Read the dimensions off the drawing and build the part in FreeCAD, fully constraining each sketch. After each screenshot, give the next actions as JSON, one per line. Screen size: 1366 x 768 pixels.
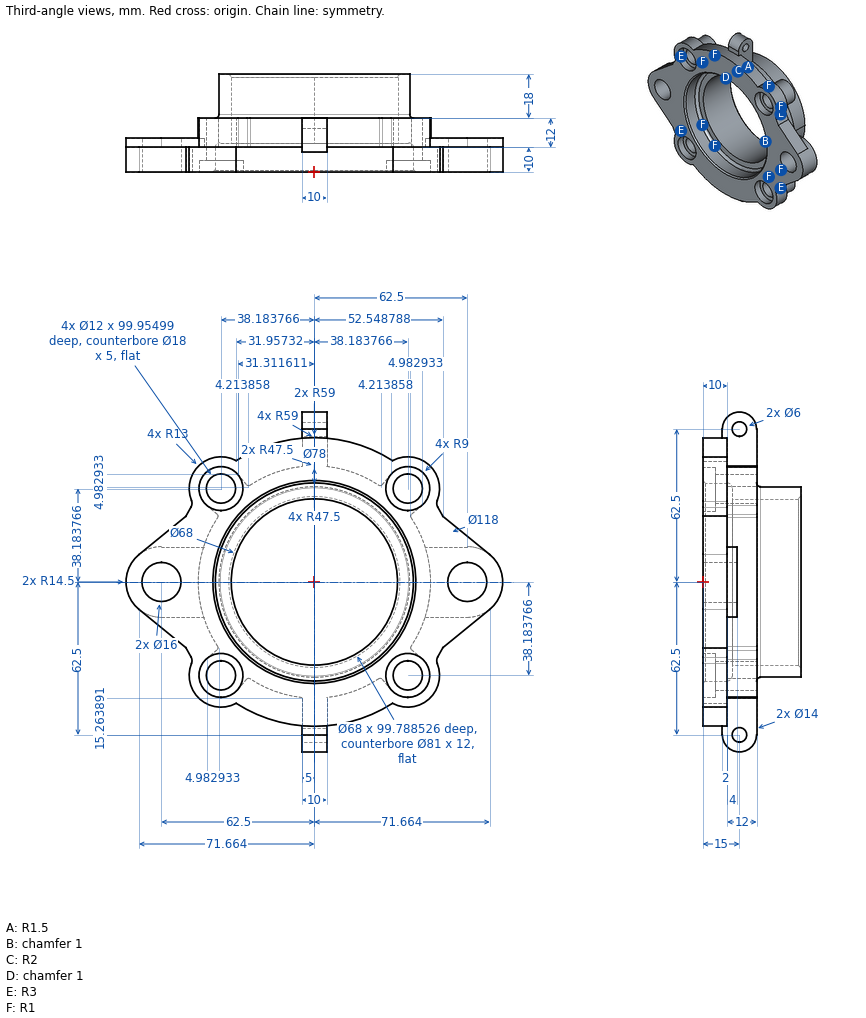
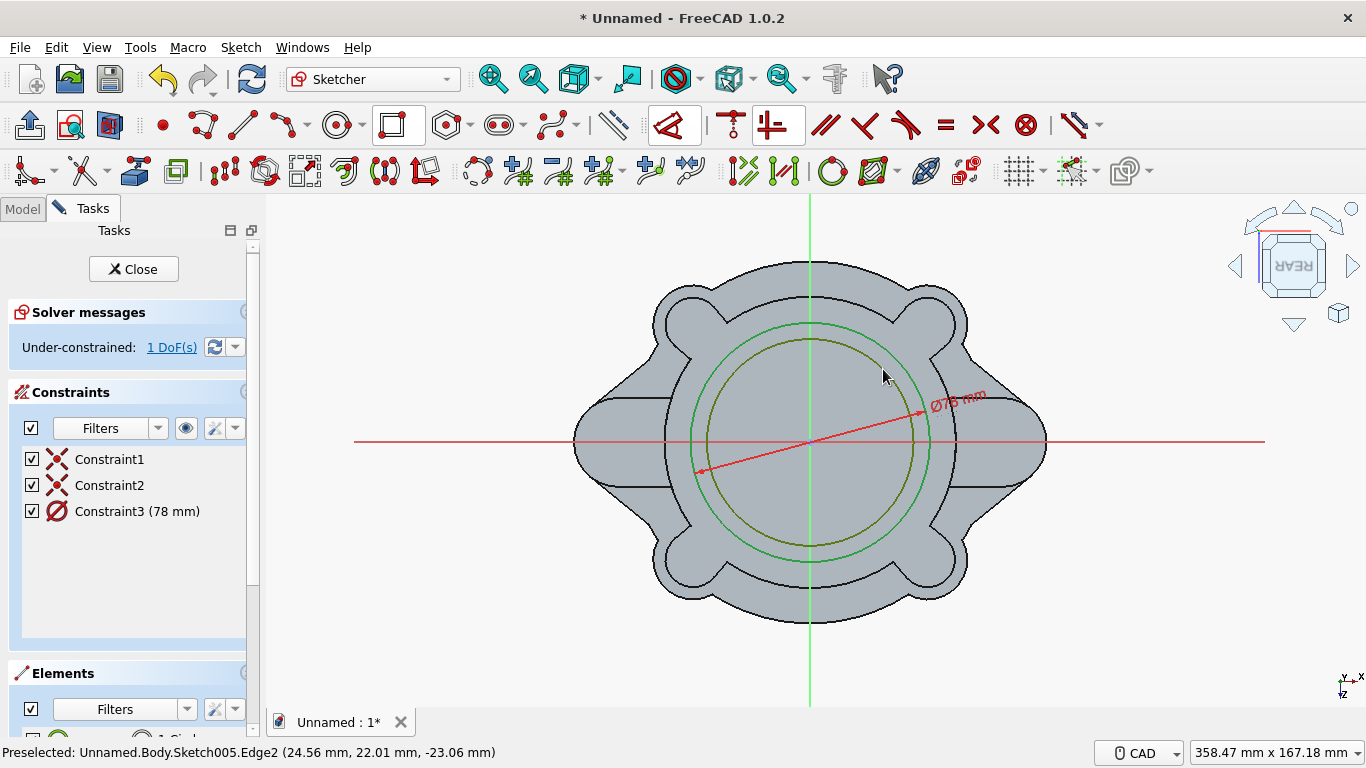
{"action": "left_click", "coordinate": [696, 126]}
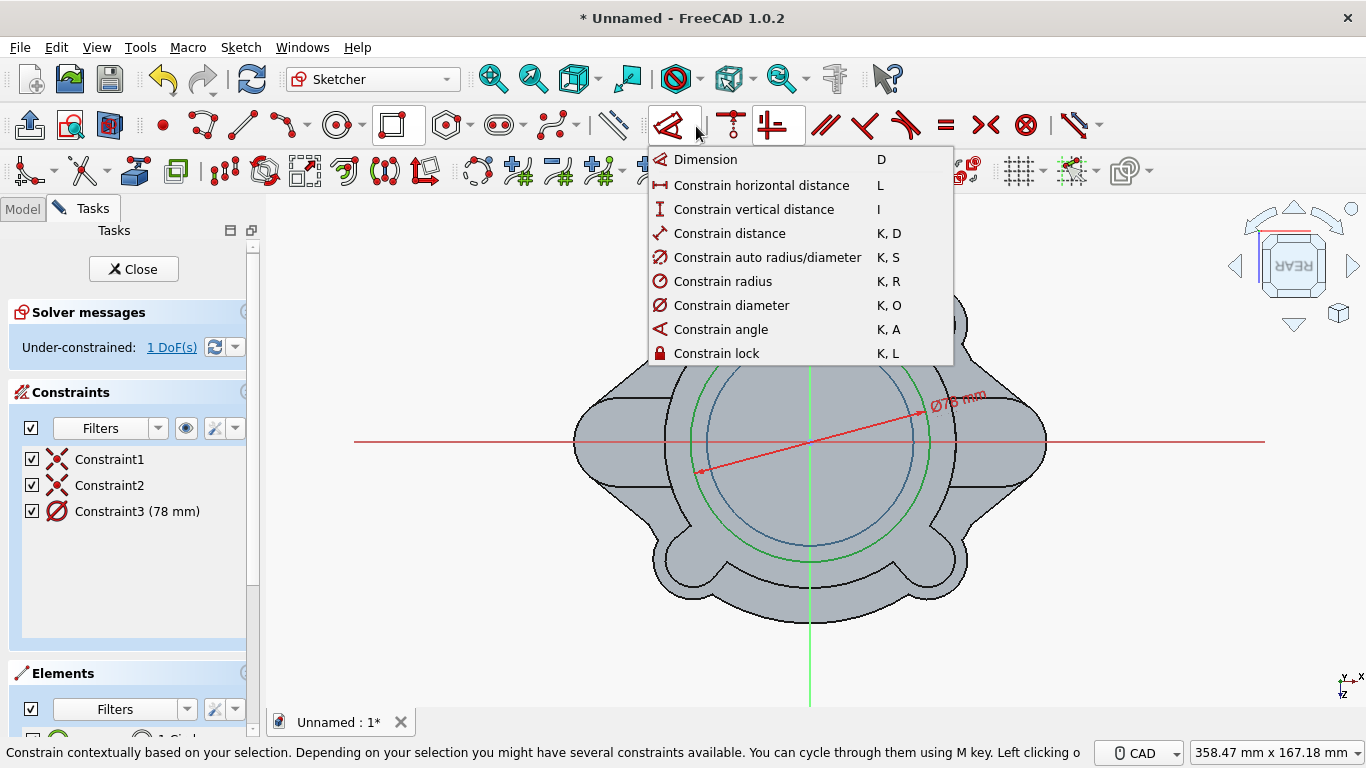
{"action": "left_click", "coordinate": [801, 305]}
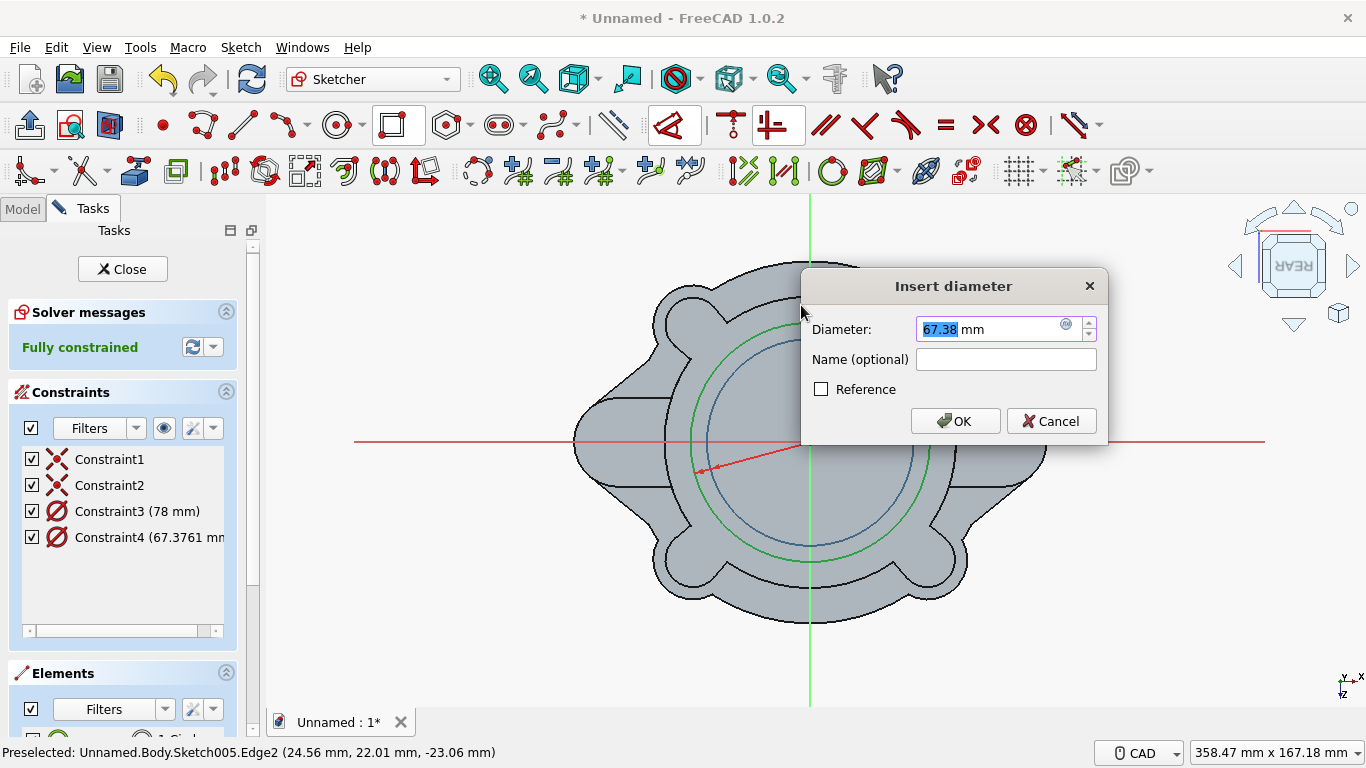
{"action": "type", "text": "68"}
{"action": "key", "text": "Return"}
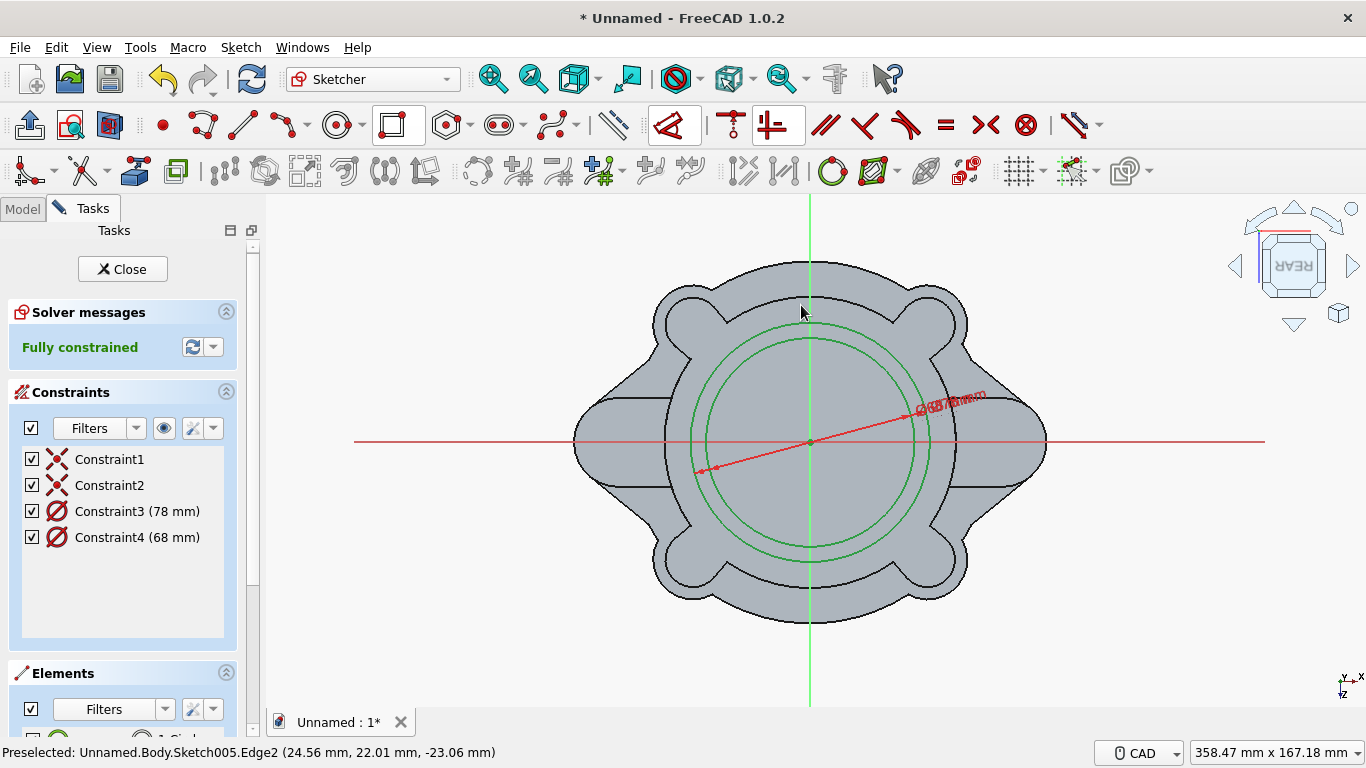
{"action": "left_click", "coordinate": [123, 269]}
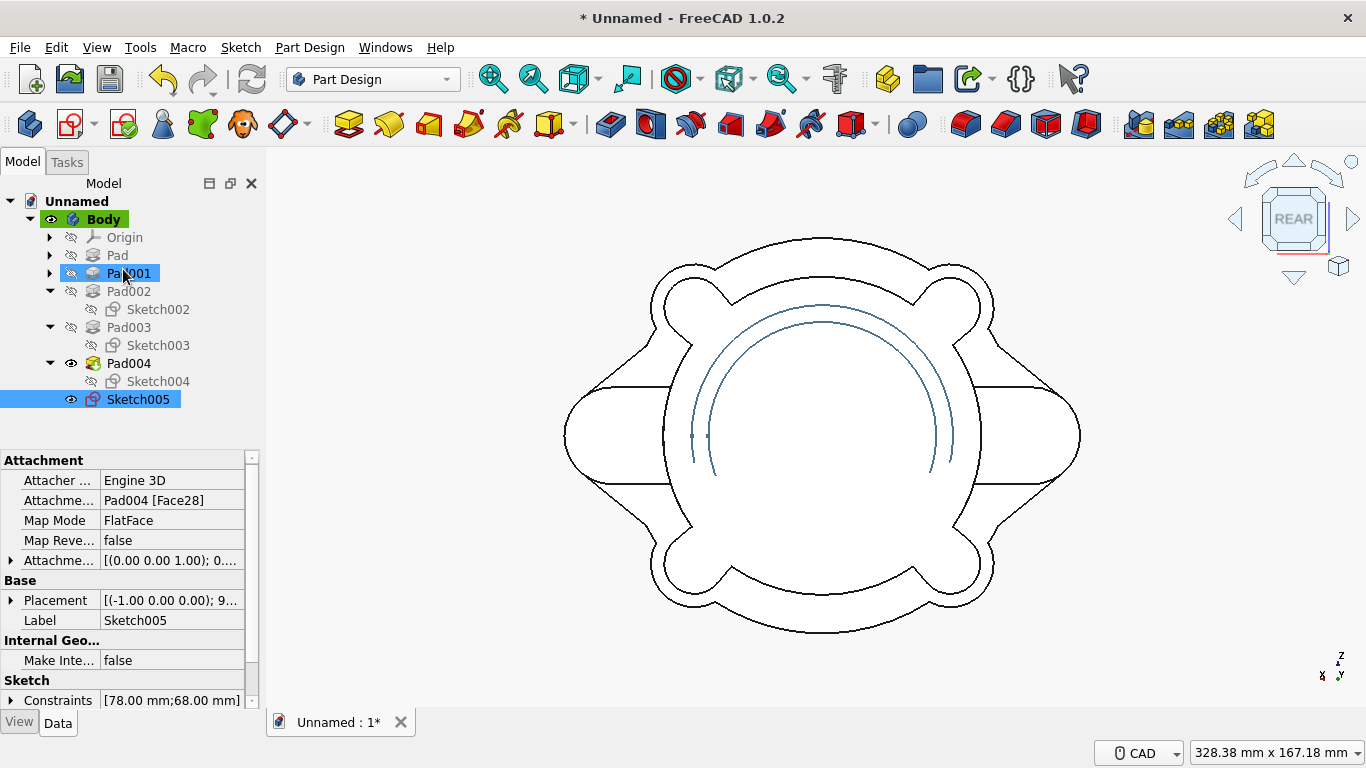
{"action": "left_click", "coordinate": [350, 124]}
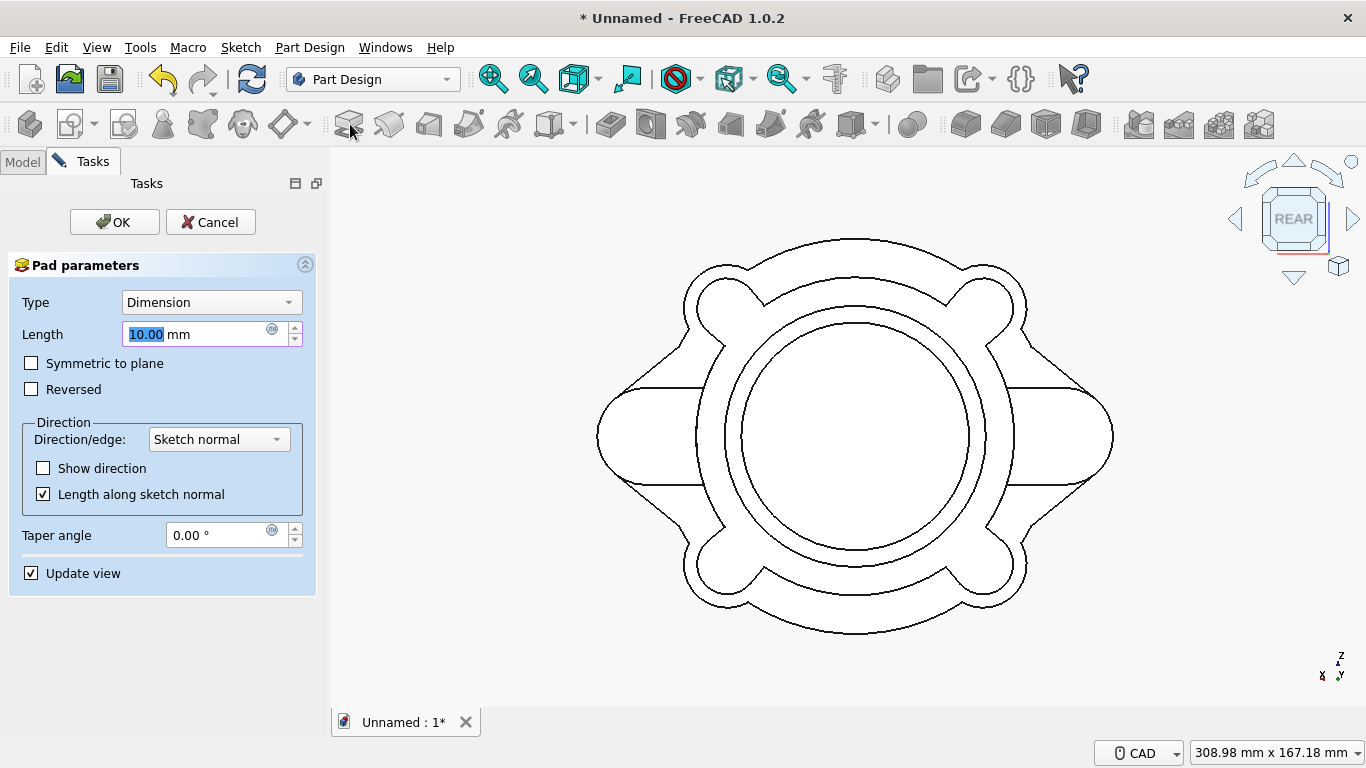
{"action": "type", "text": "18"}
{"action": "key", "text": "Tab"}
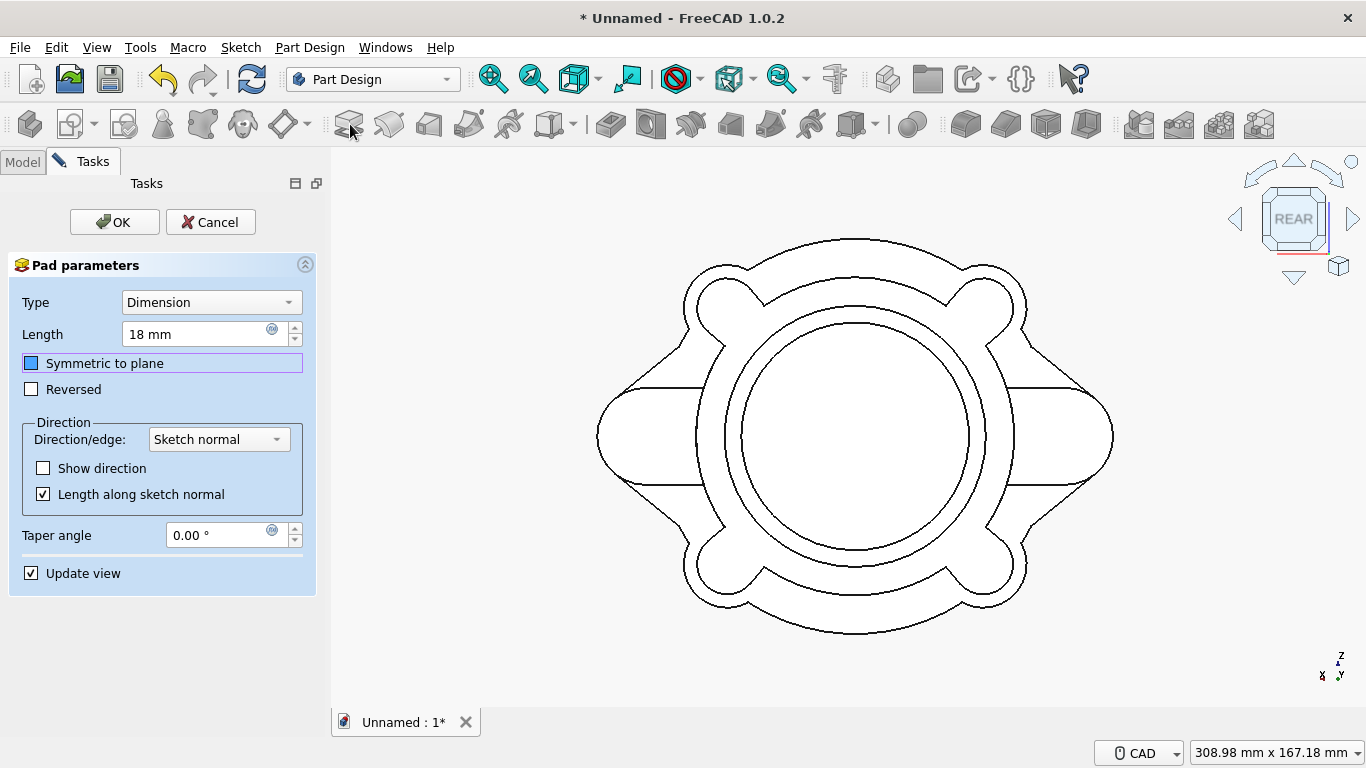
{"action": "left_click", "coordinate": [115, 222]}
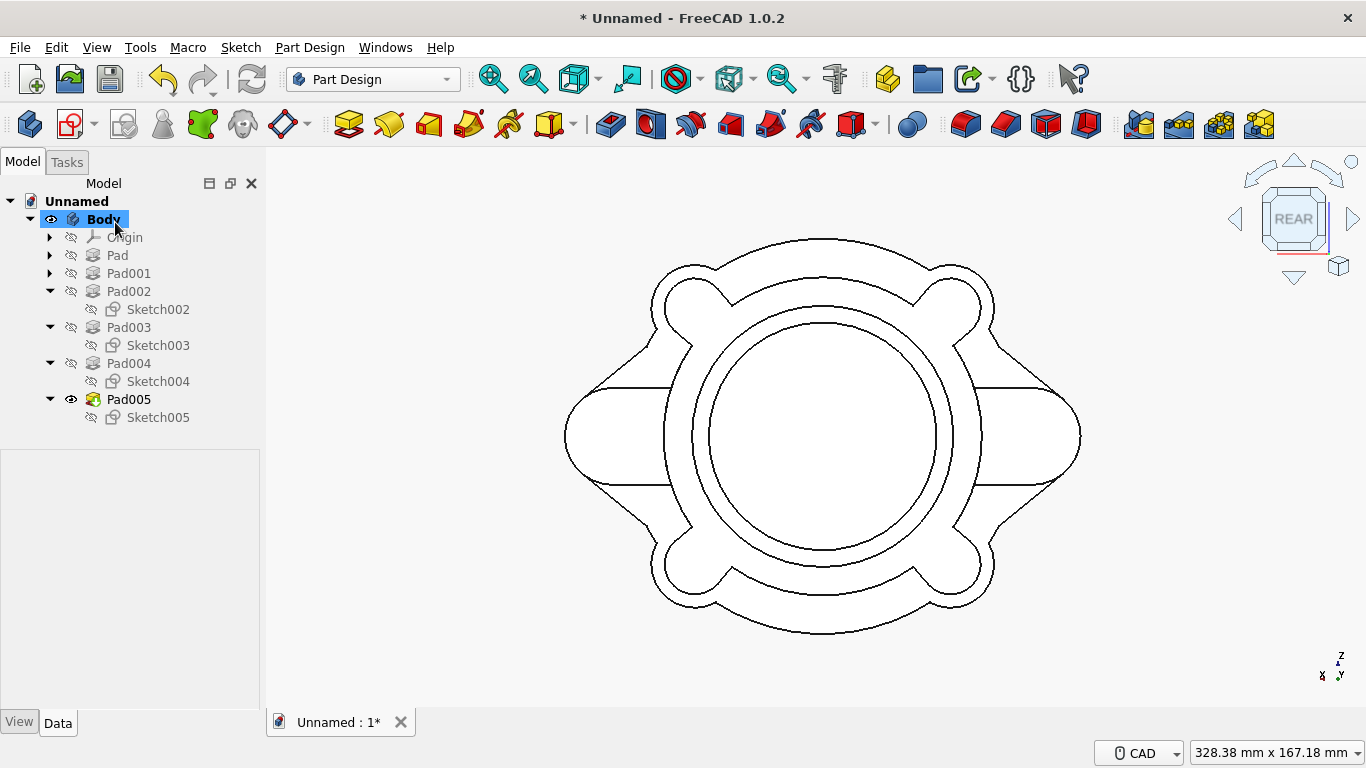
{"action": "key", "text": "0"}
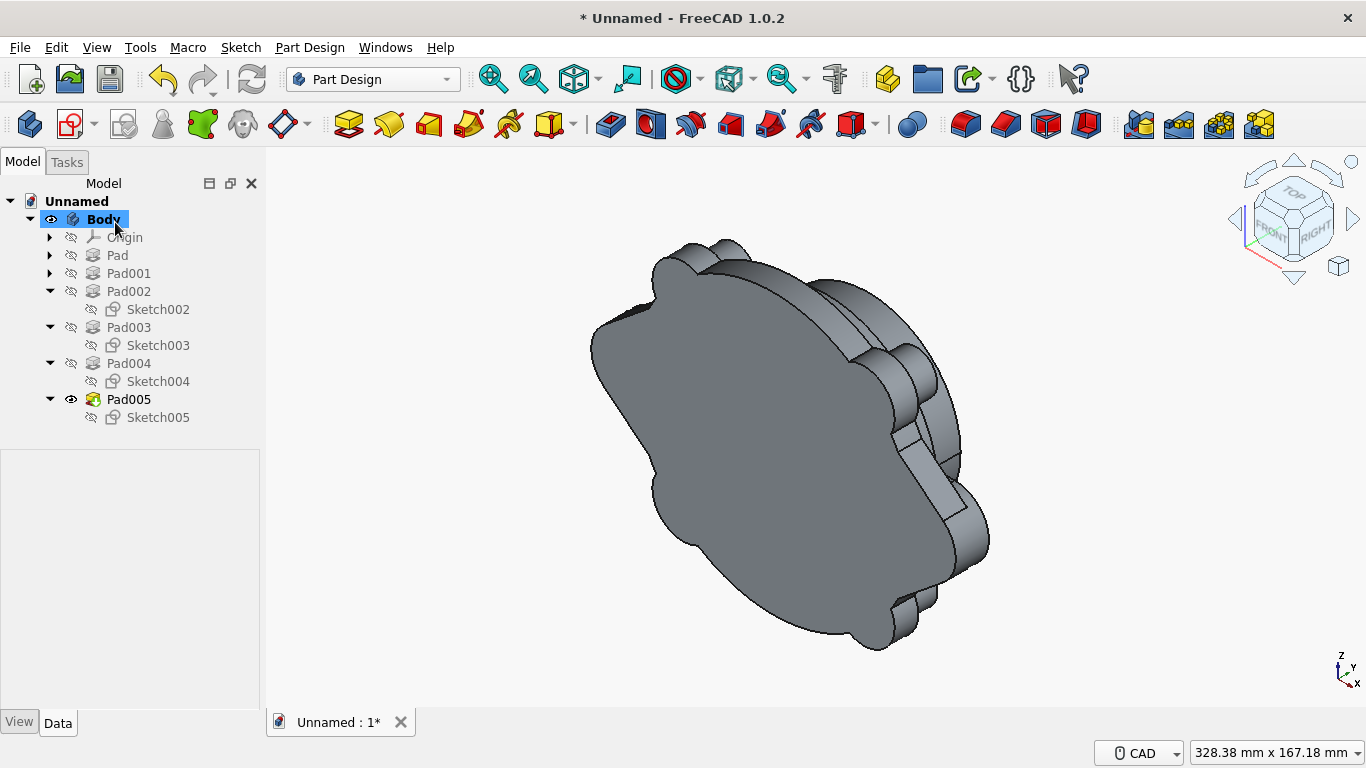
{"action": "left_click", "coordinate": [494, 80]}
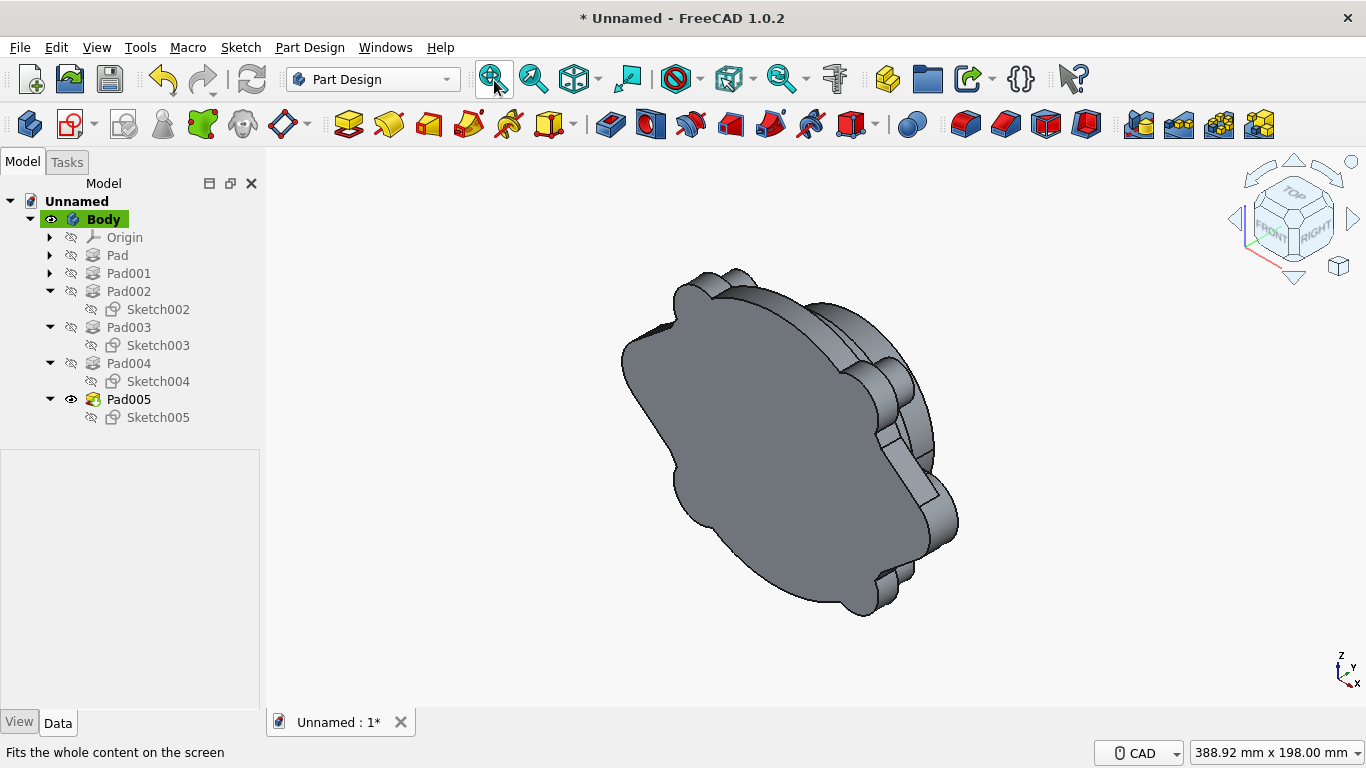
{"action": "key", "text": "2"}